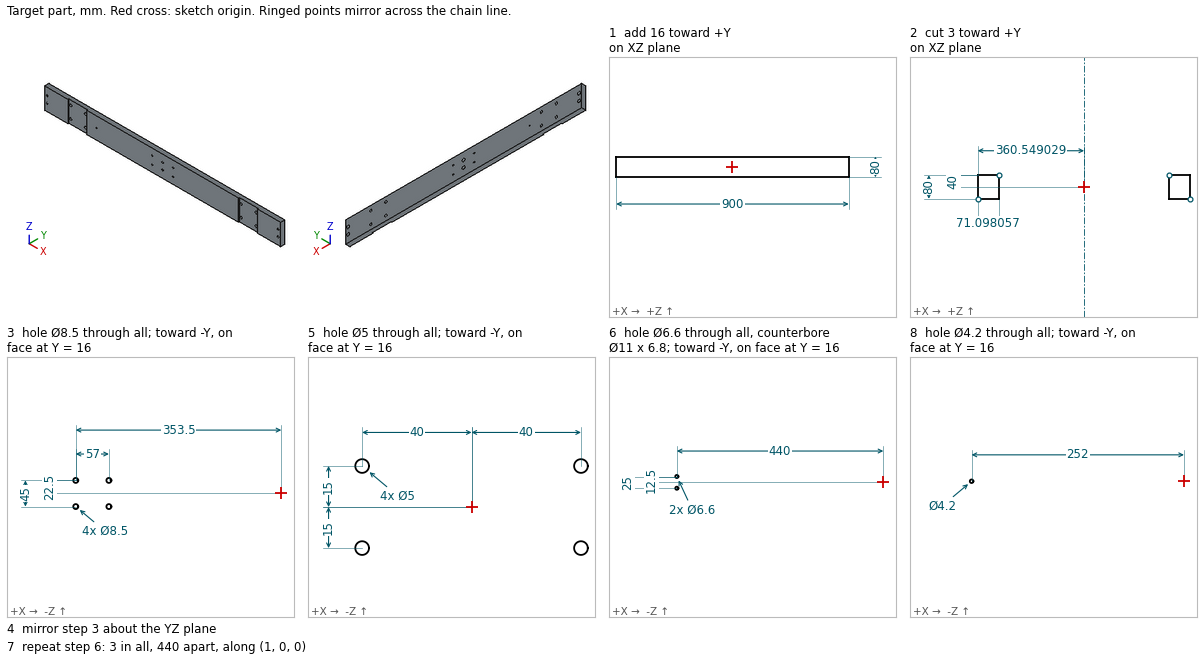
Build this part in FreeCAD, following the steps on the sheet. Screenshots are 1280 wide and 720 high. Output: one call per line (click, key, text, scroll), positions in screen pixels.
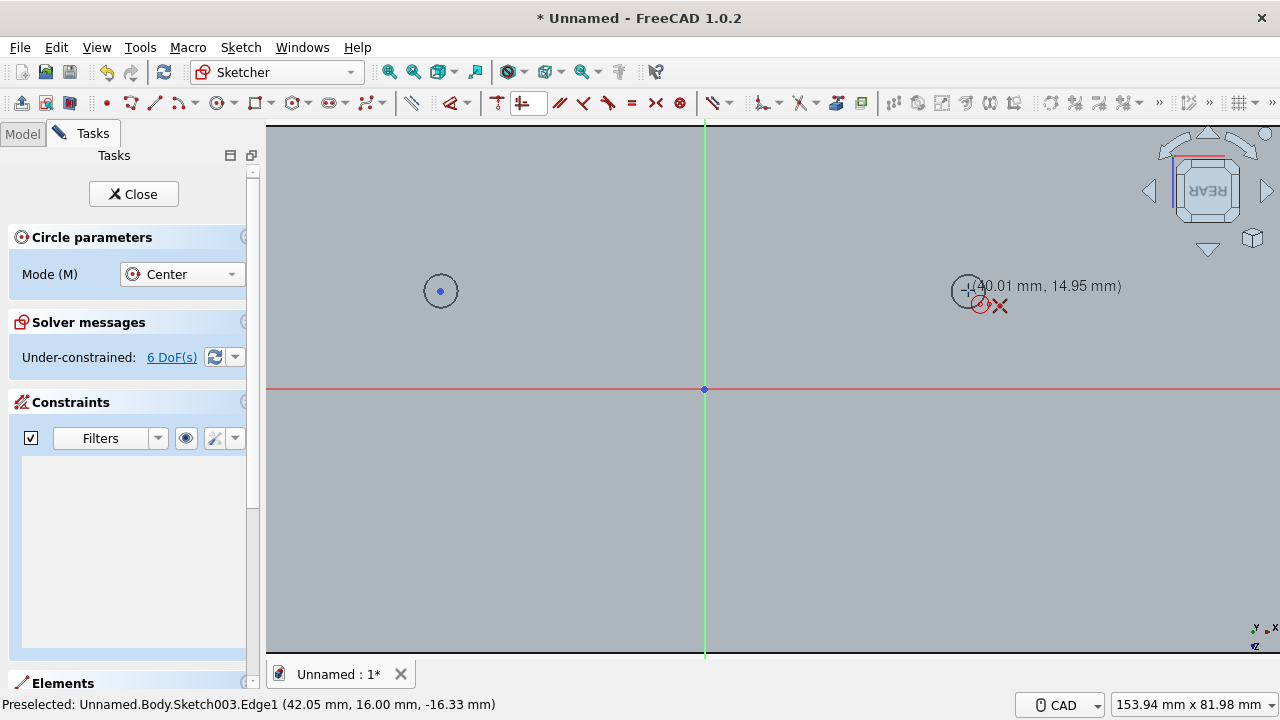
scroll(441, 488, up, 2)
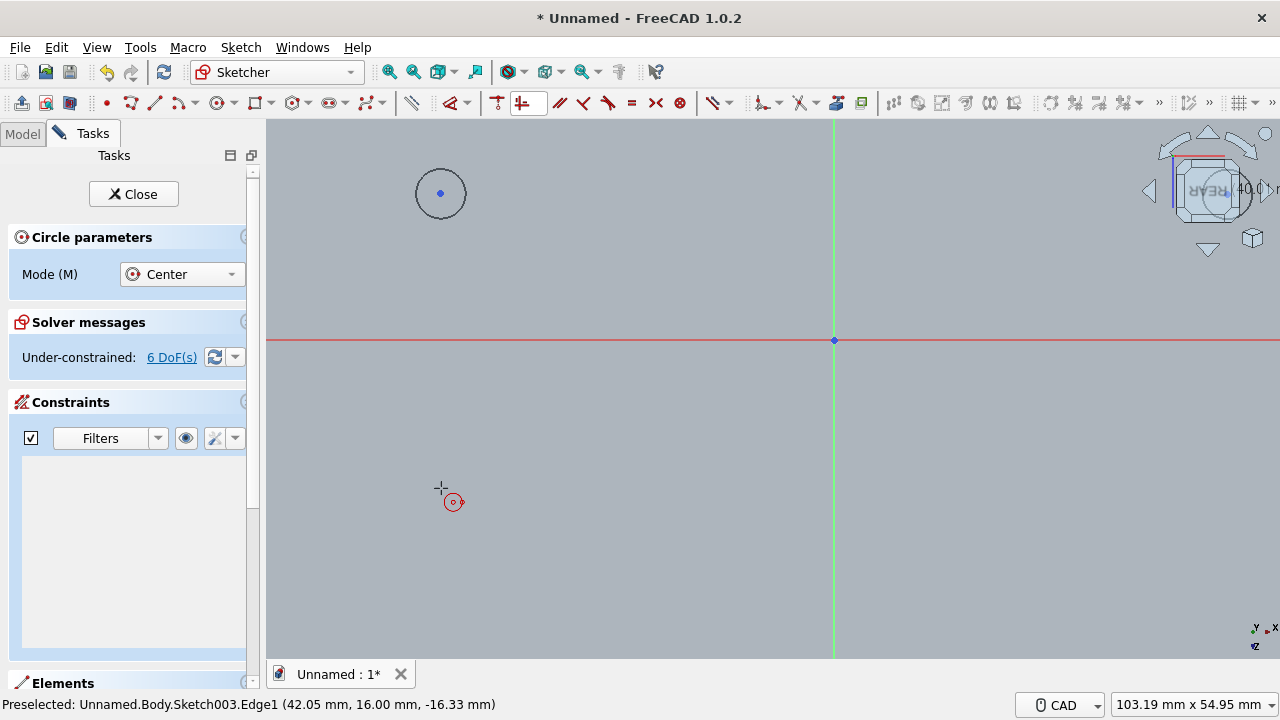
click(441, 488)
click(459, 470)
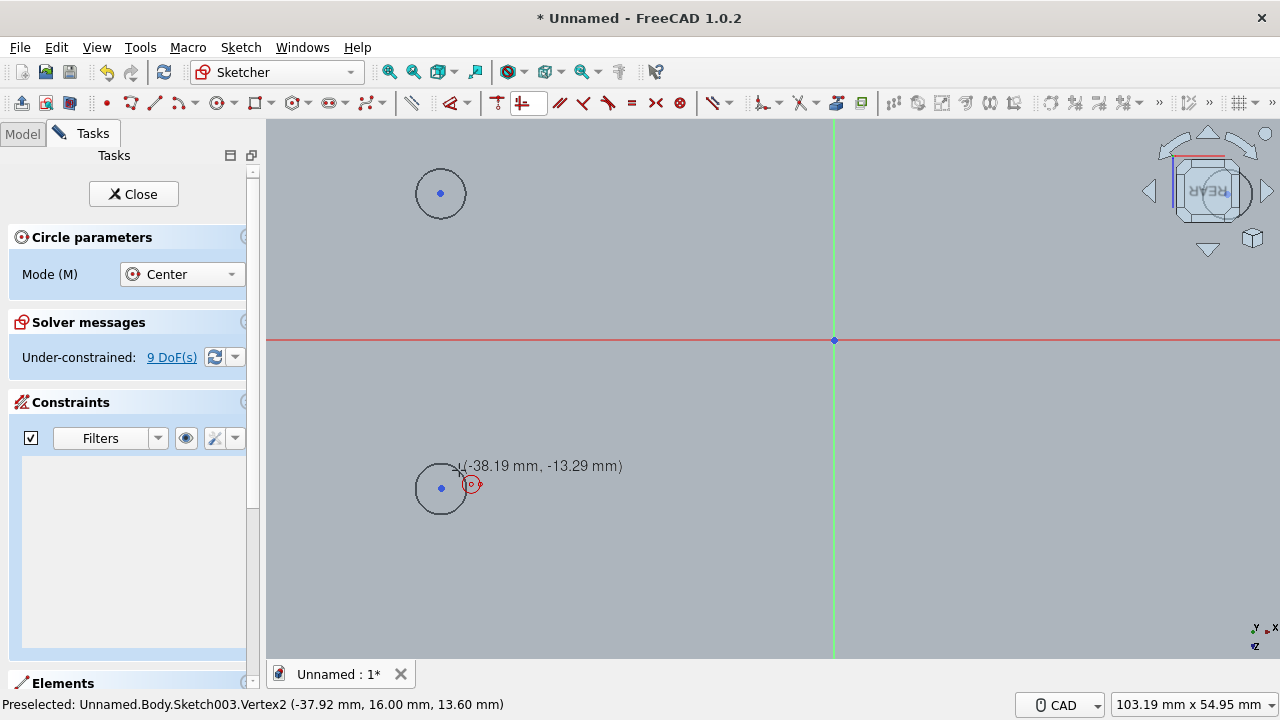
scroll(441, 488, down, 2)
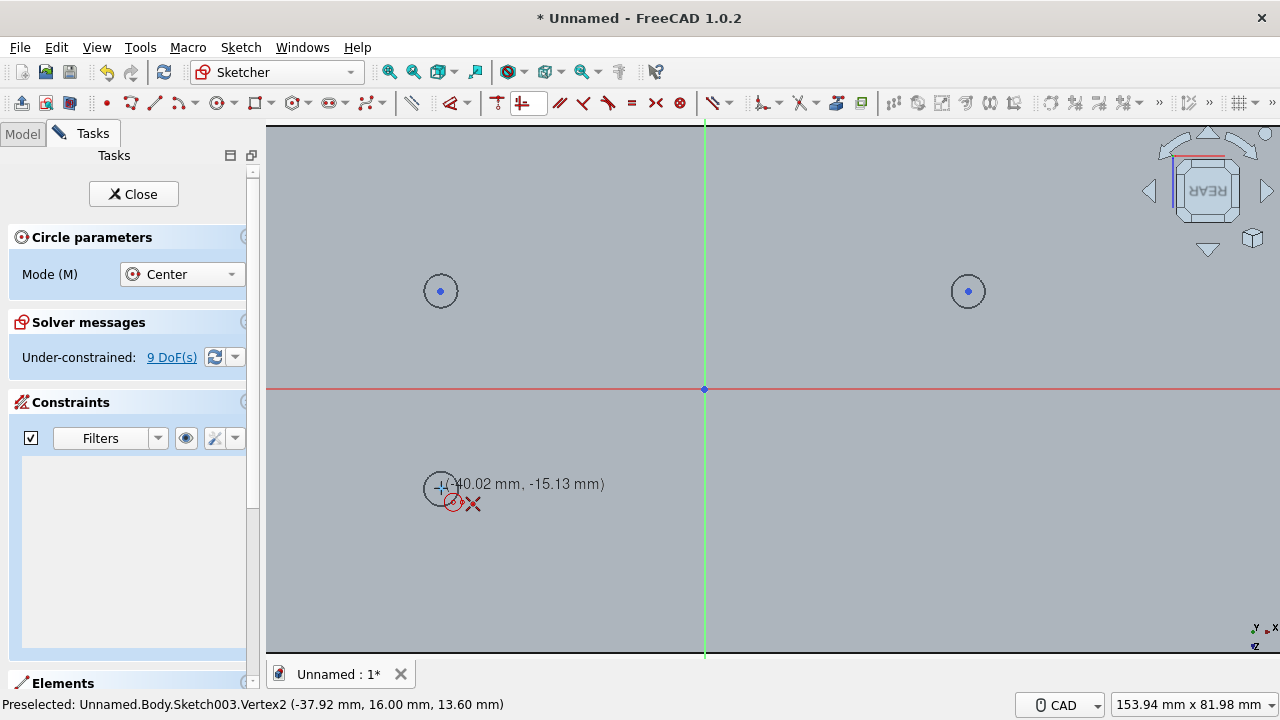
scroll(968, 488, up, 2)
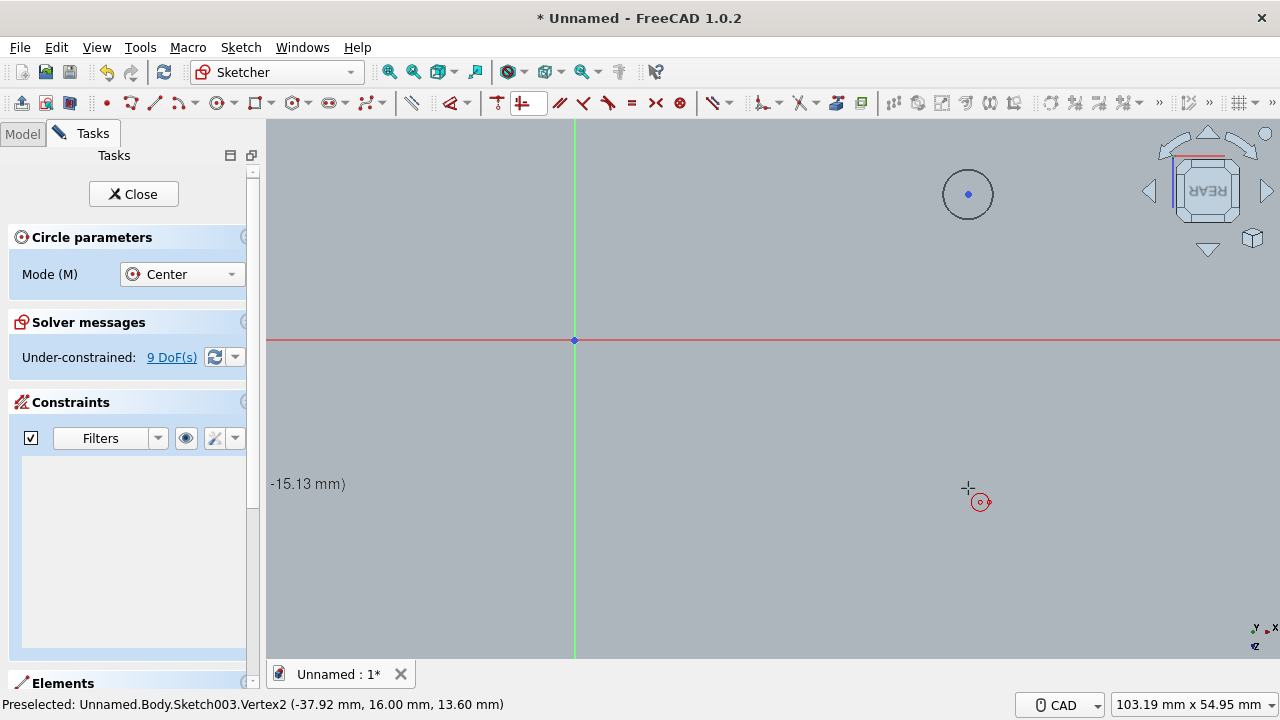
click(968, 488)
click(985, 470)
key(Escape)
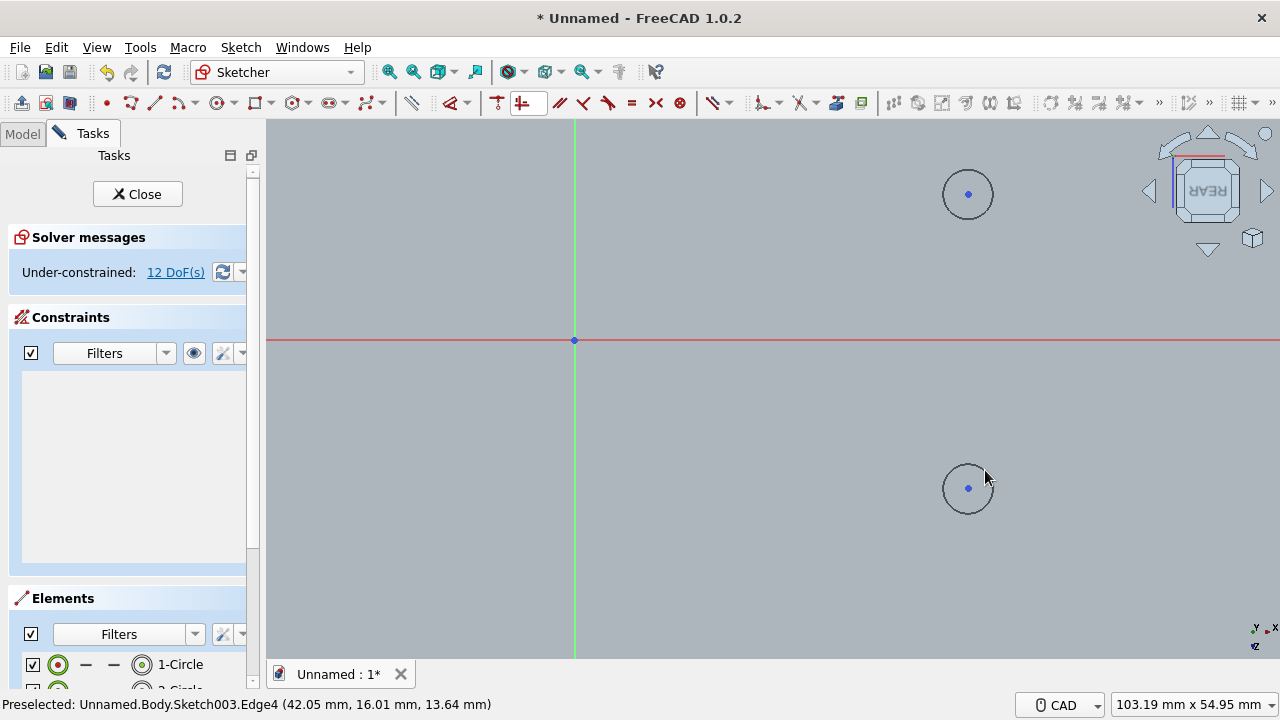
scroll(968, 488, down, 2)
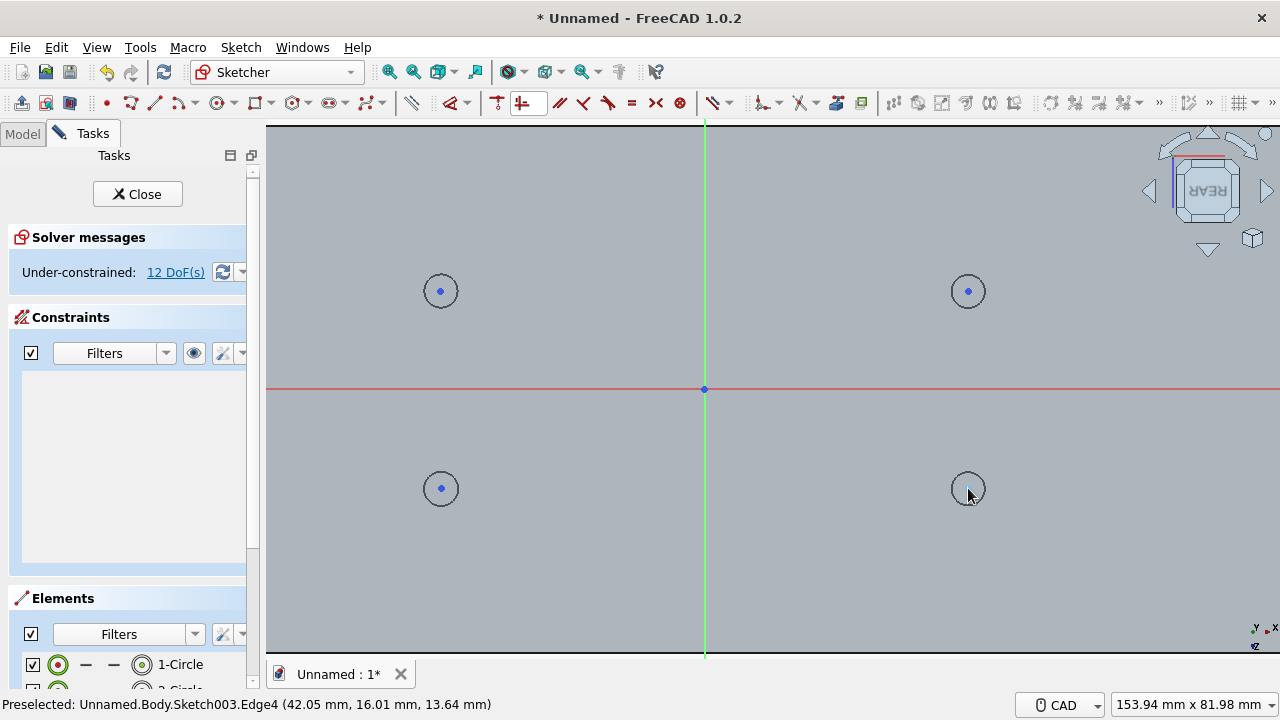
click(453, 279)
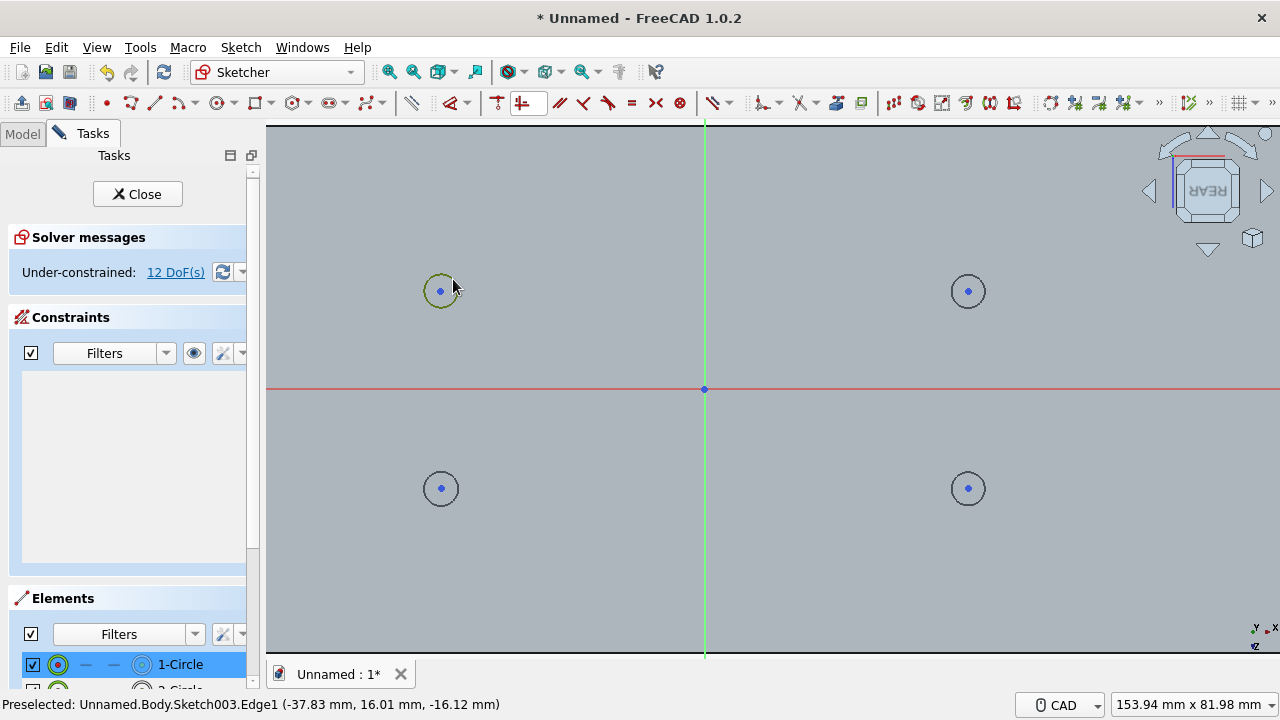
click(980, 280)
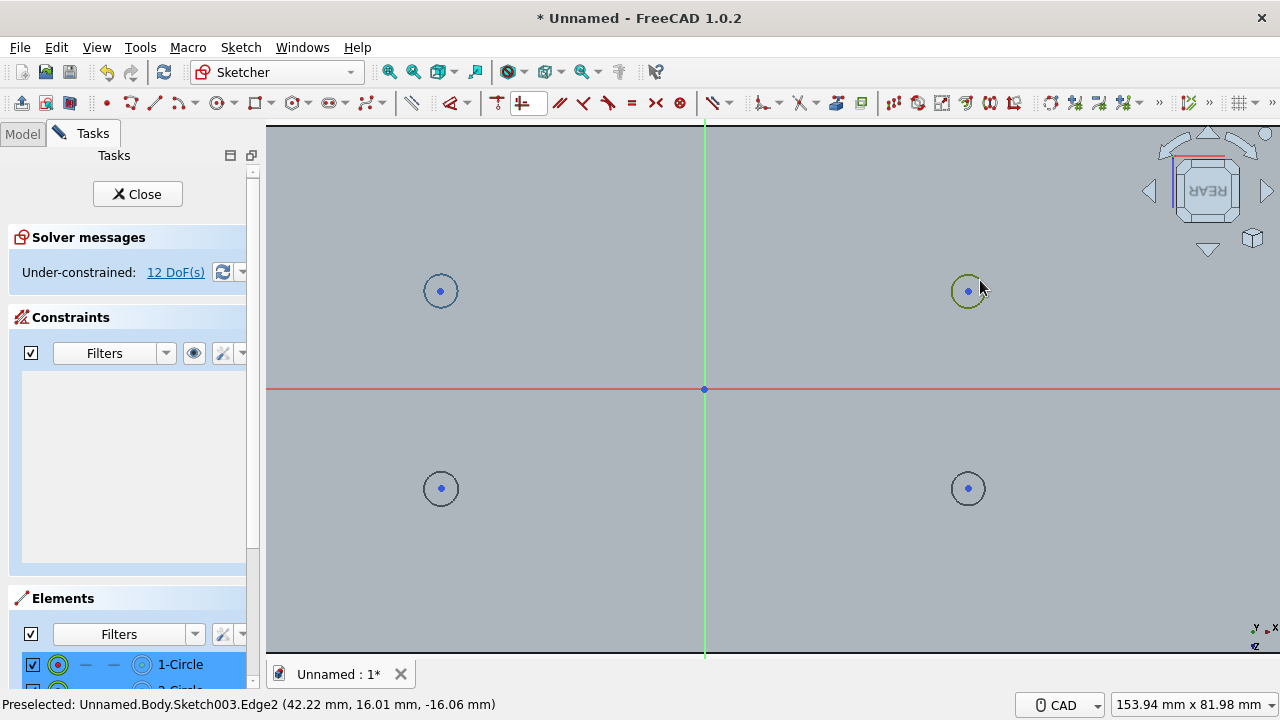
click(453, 477)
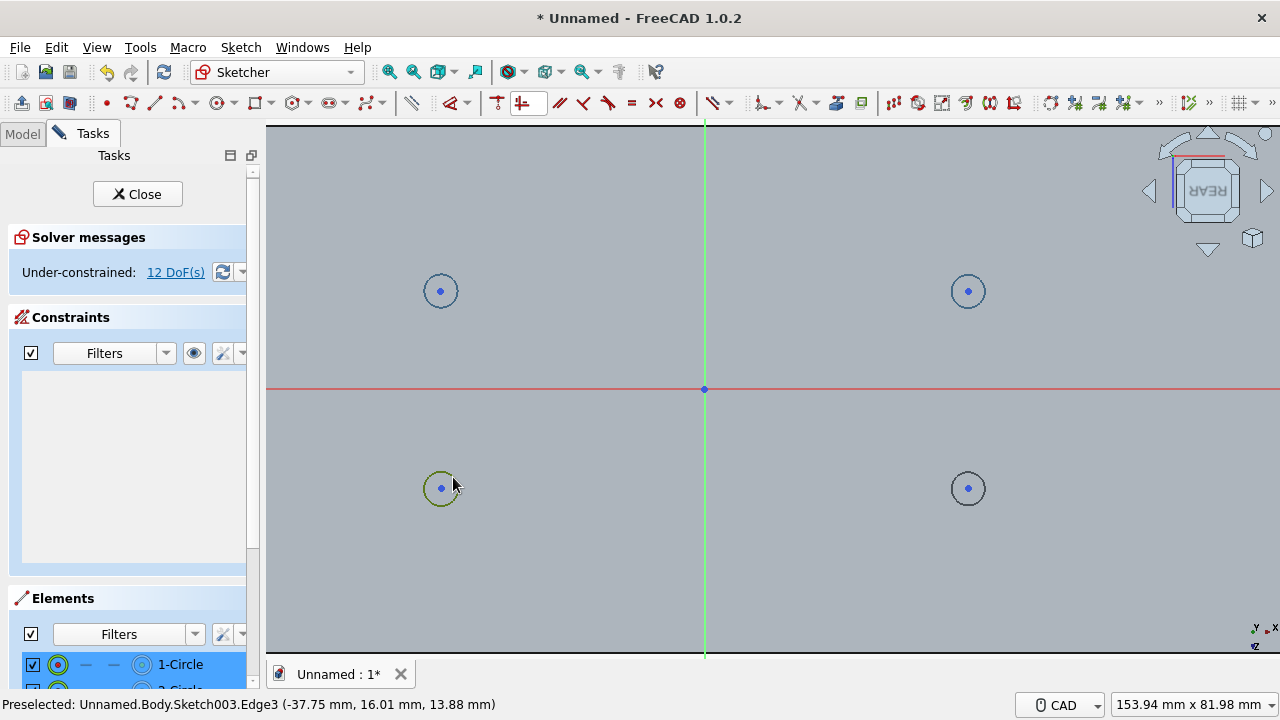
click(980, 477)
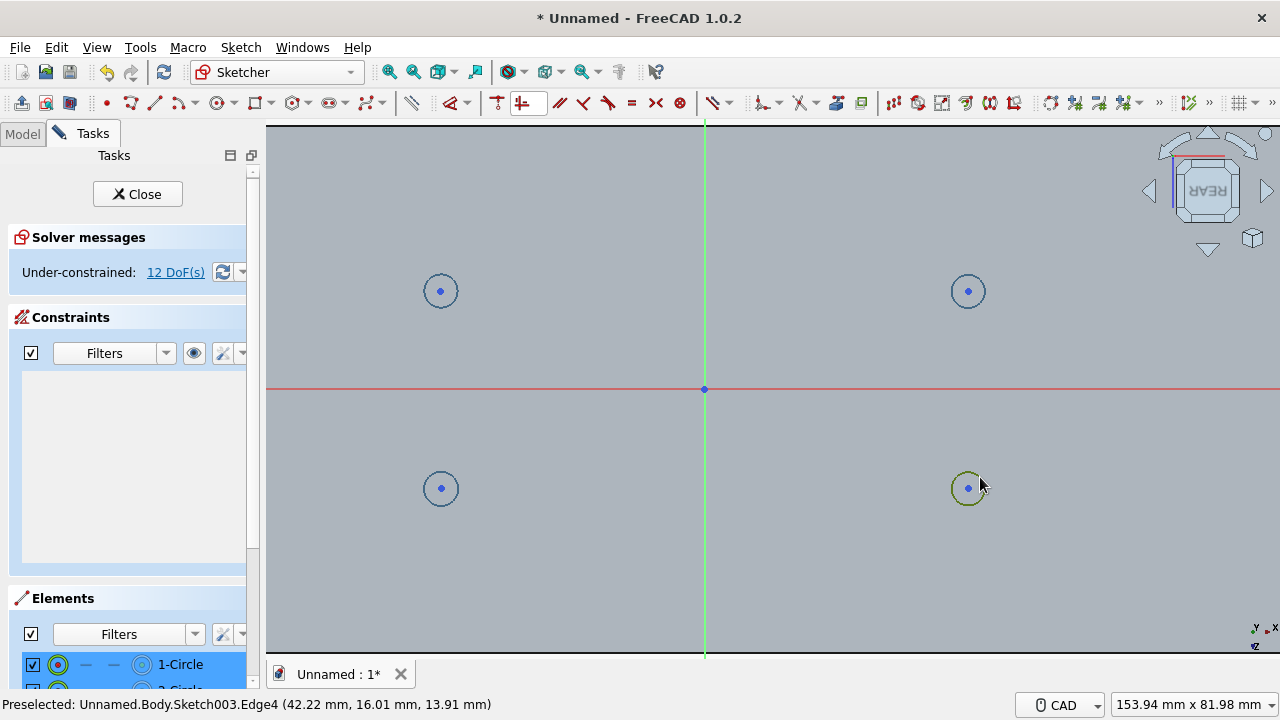
click(632, 104)